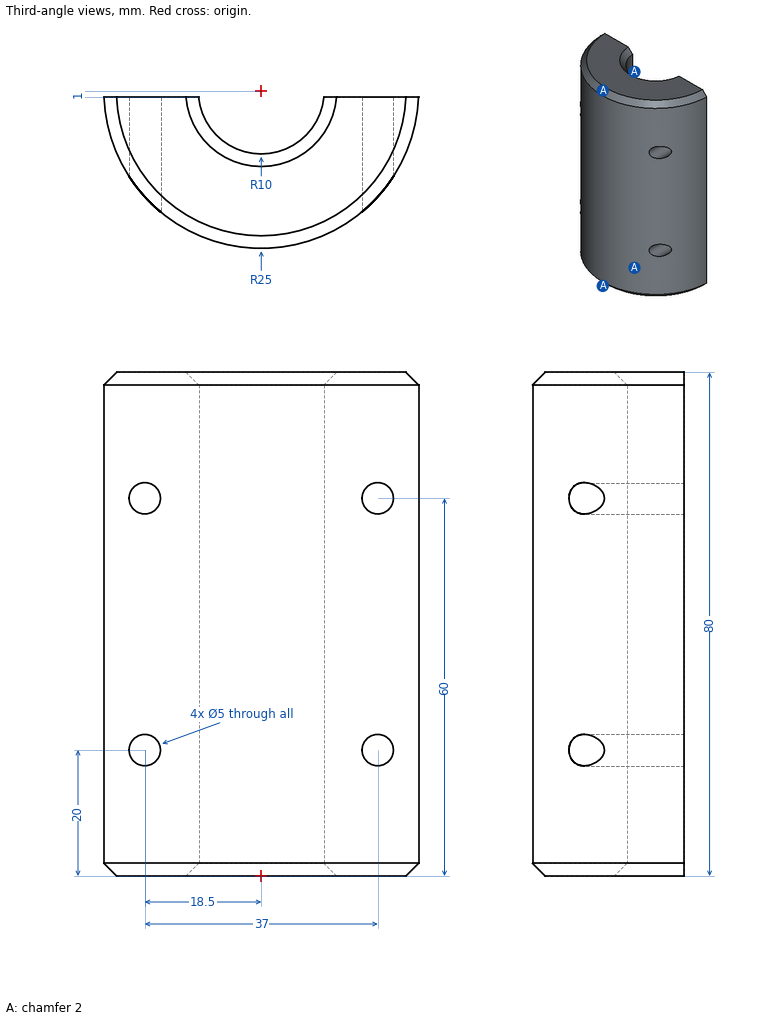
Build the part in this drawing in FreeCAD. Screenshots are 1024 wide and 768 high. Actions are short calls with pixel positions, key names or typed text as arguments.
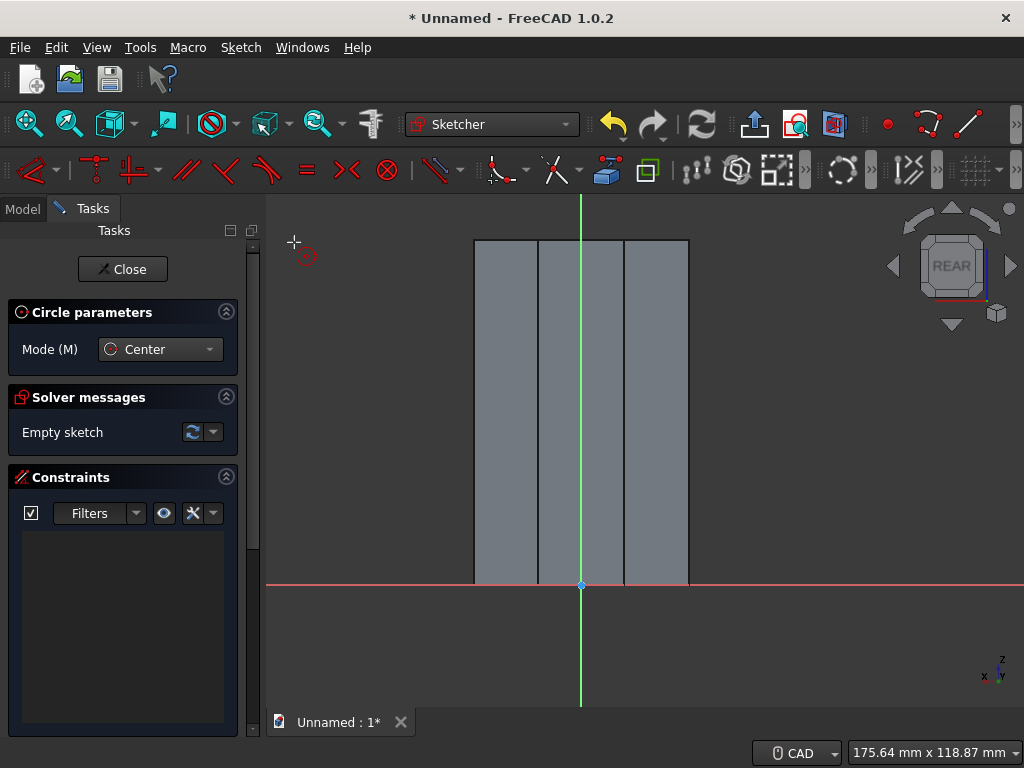
scroll(661, 499, up, 4)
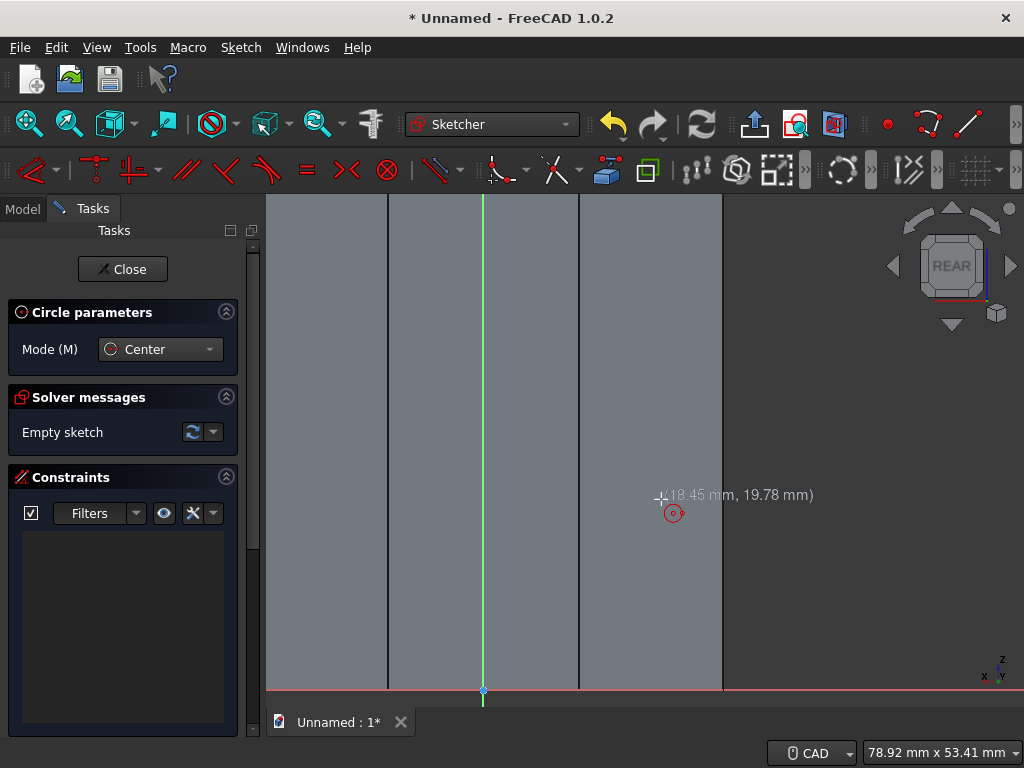
click(661, 498)
click(678, 481)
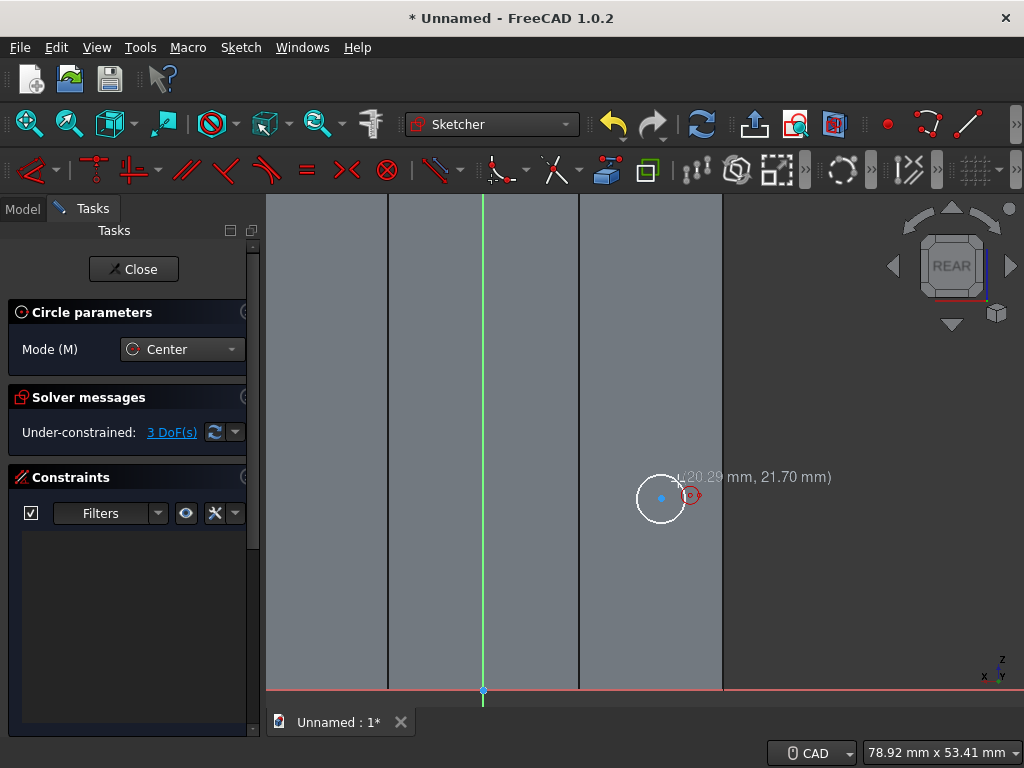
click(305, 498)
click(322, 481)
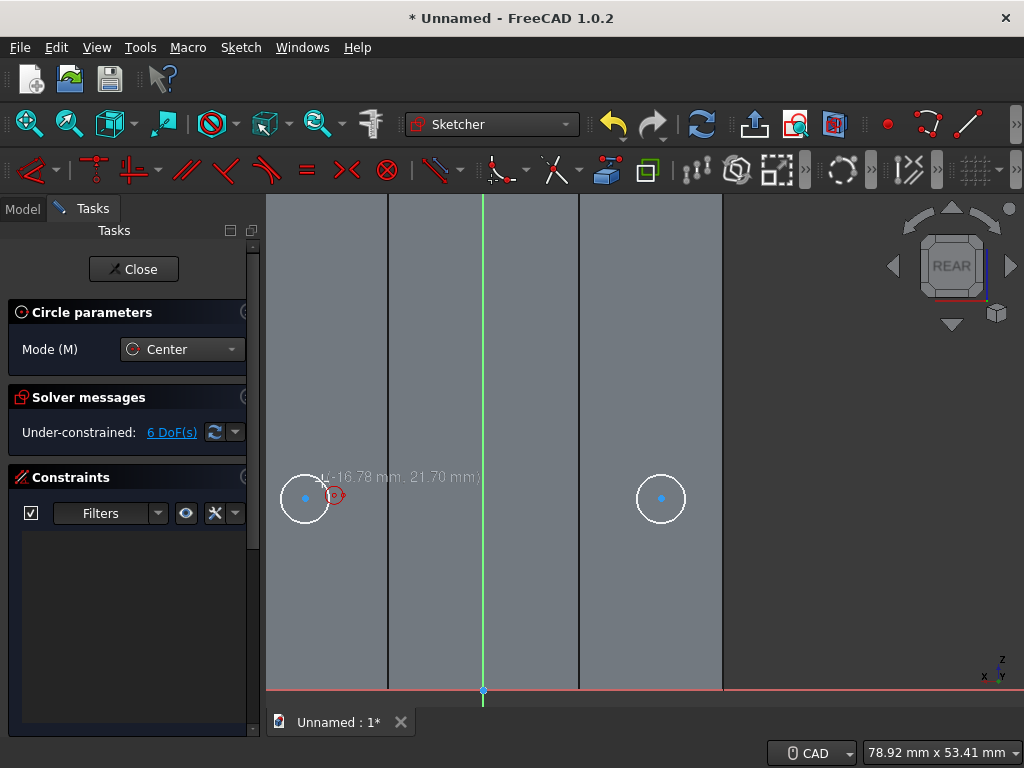
scroll(690, 524, down, 3)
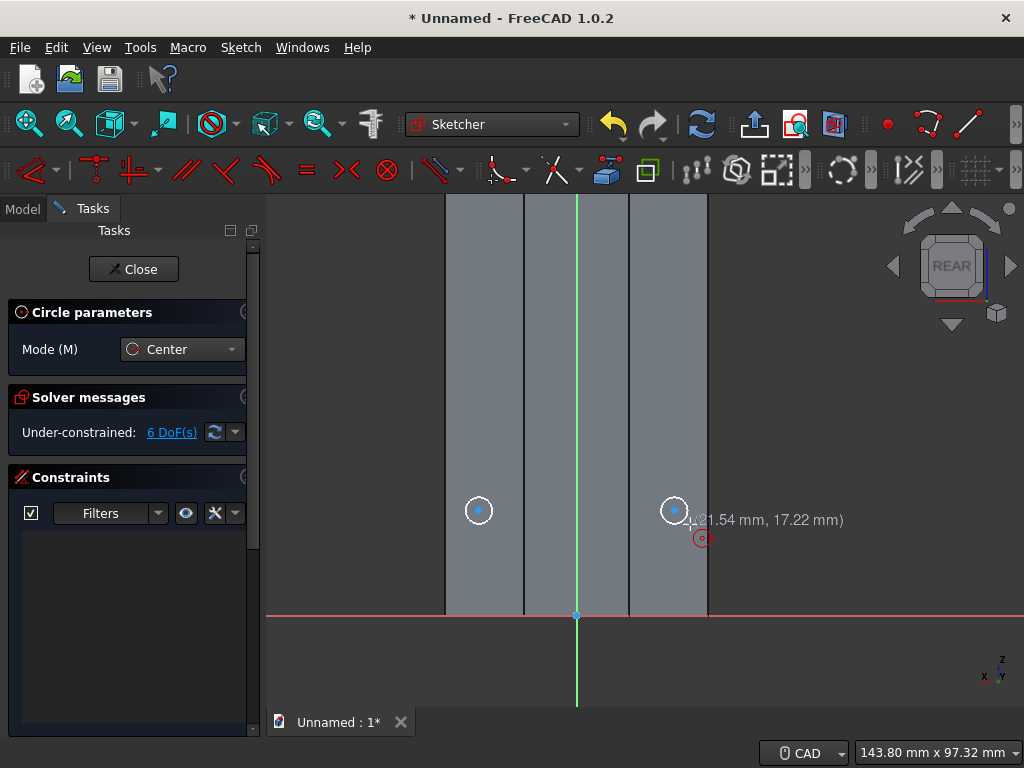
scroll(479, 299, up, 3)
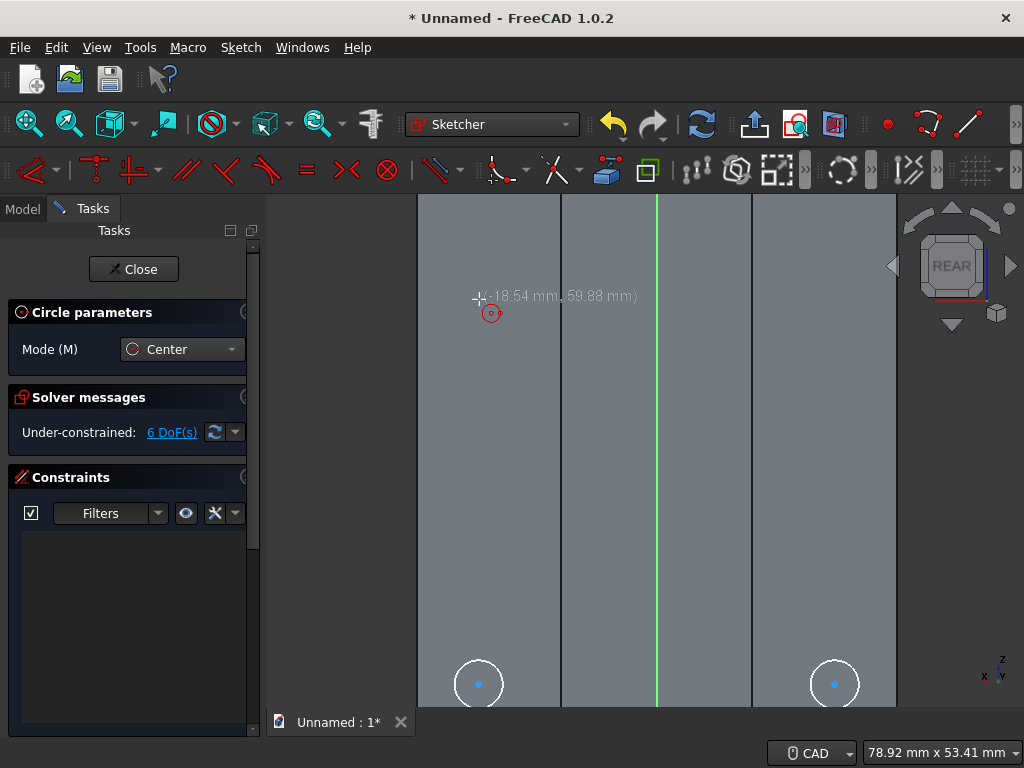
click(479, 300)
click(496, 283)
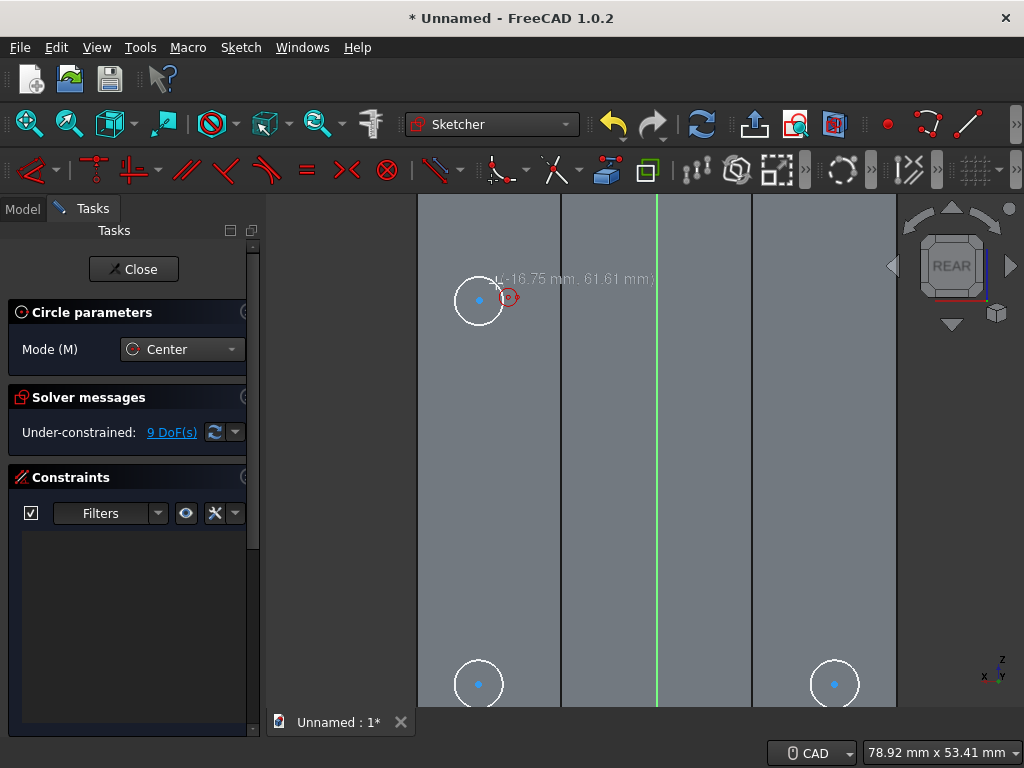
click(835, 300)
click(852, 283)
key(Escape)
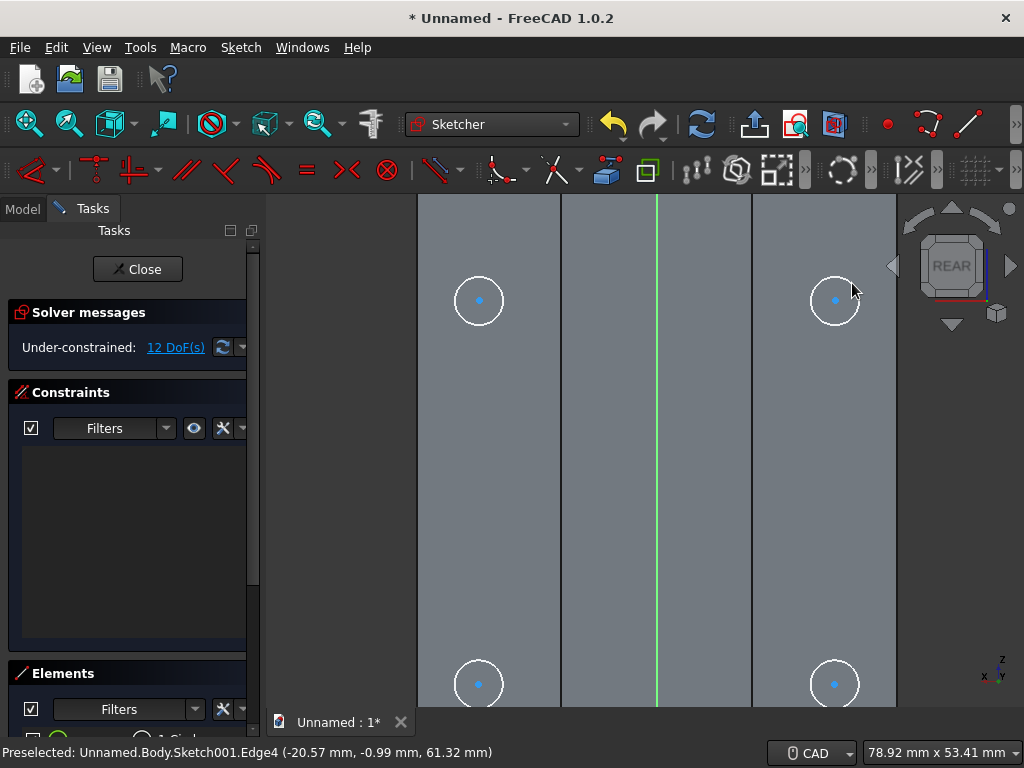
click(852, 667)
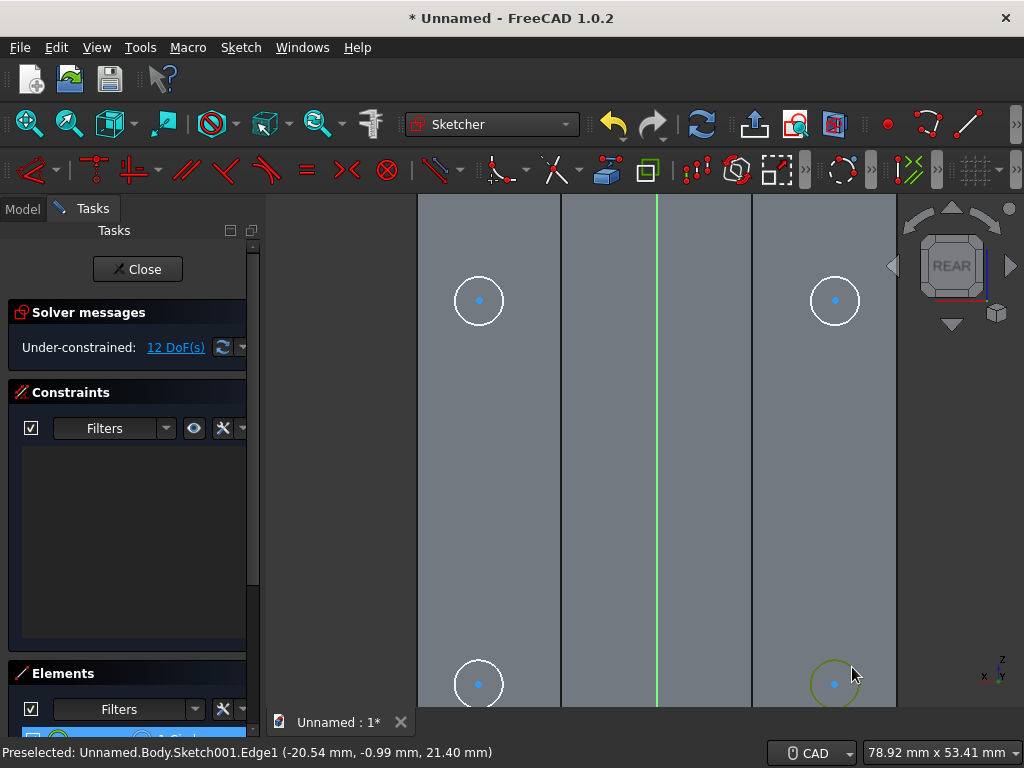
click(496, 667)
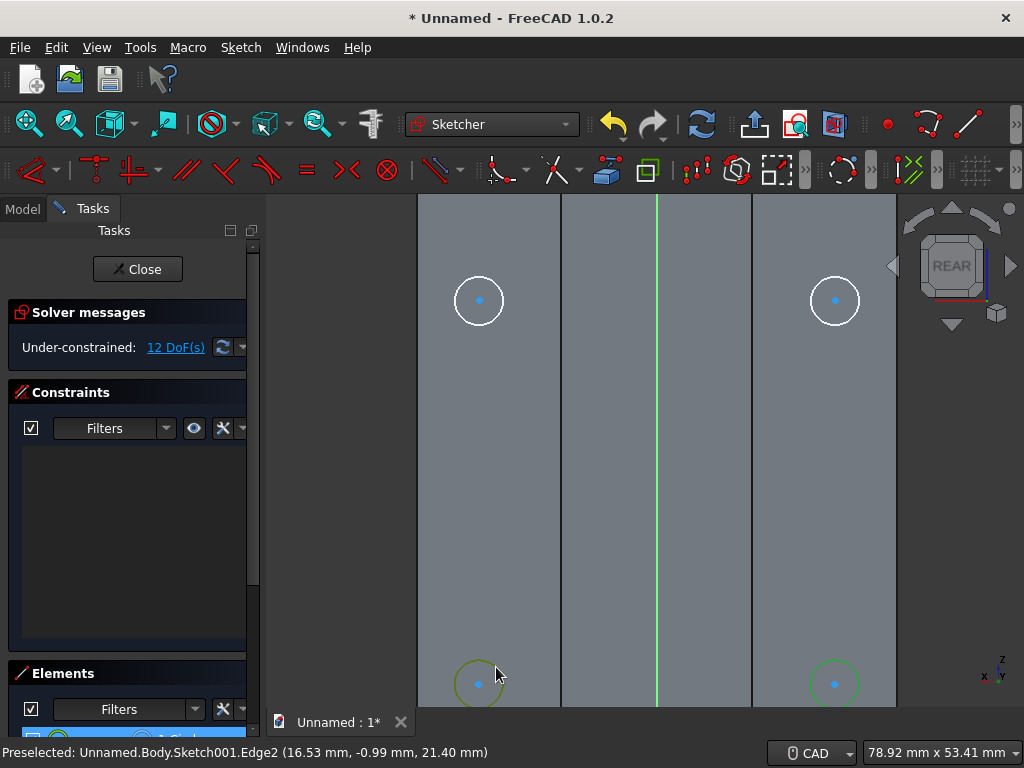
click(496, 284)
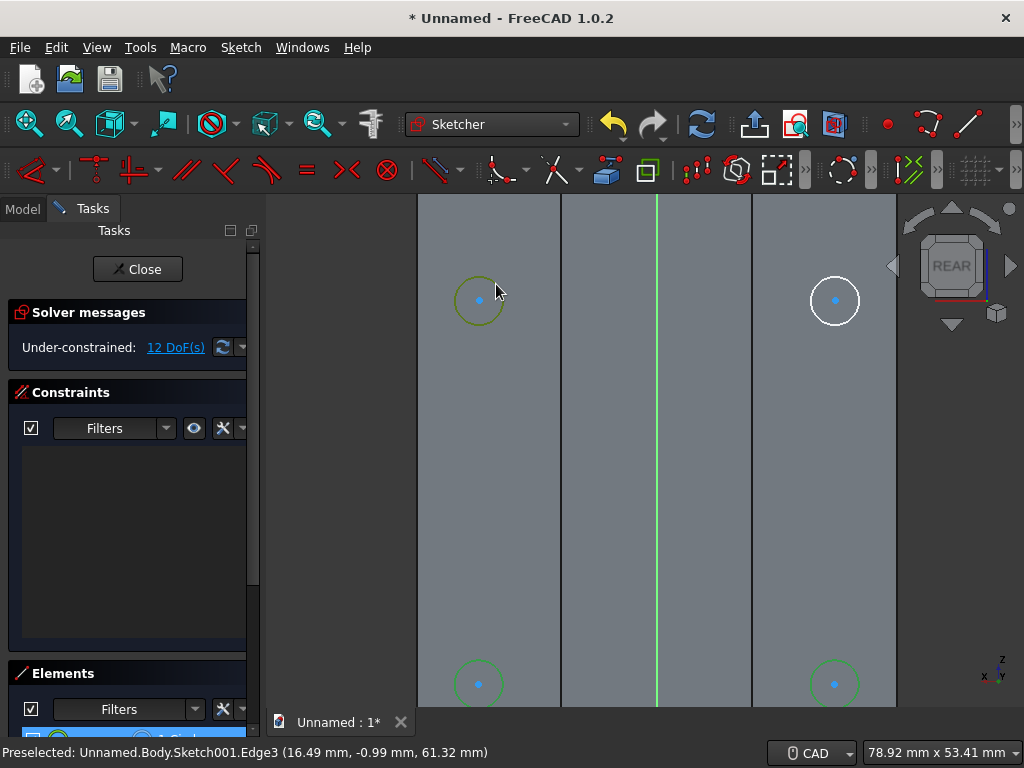
click(852, 284)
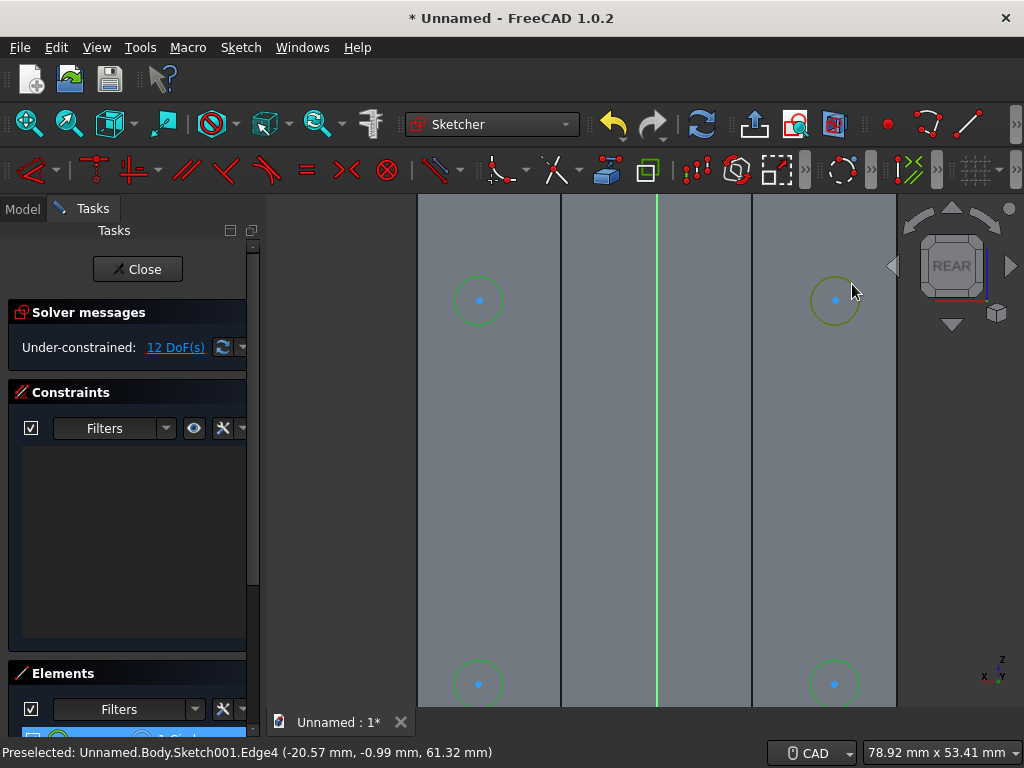
key(e)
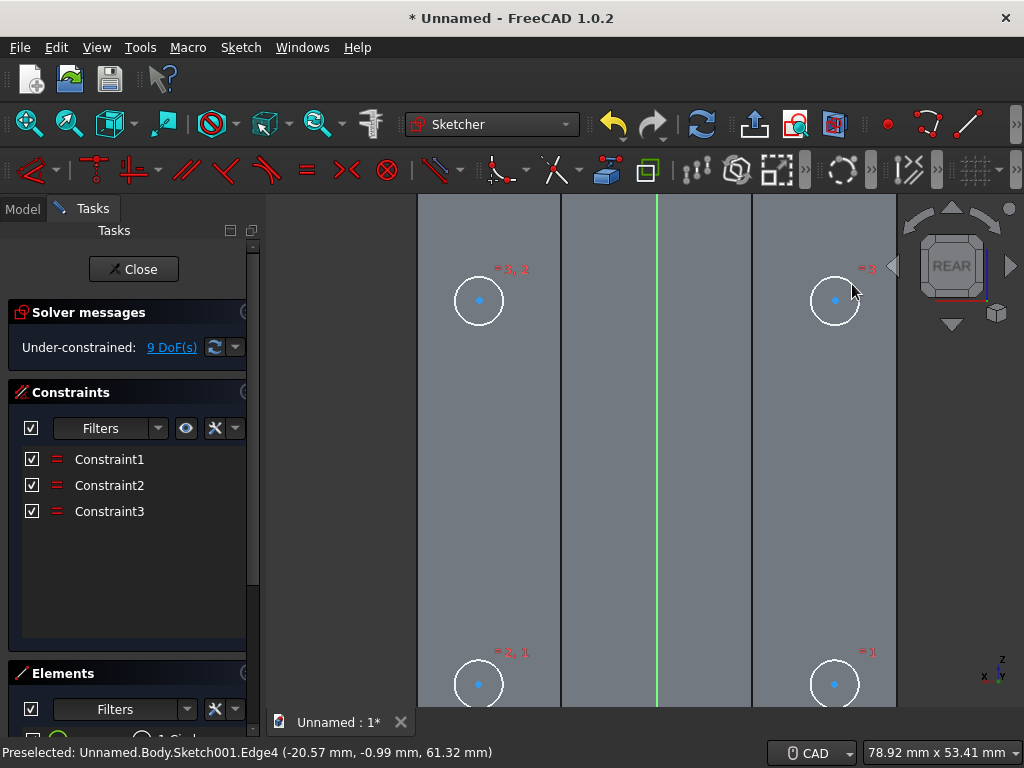
scroll(479, 298, down, 3)